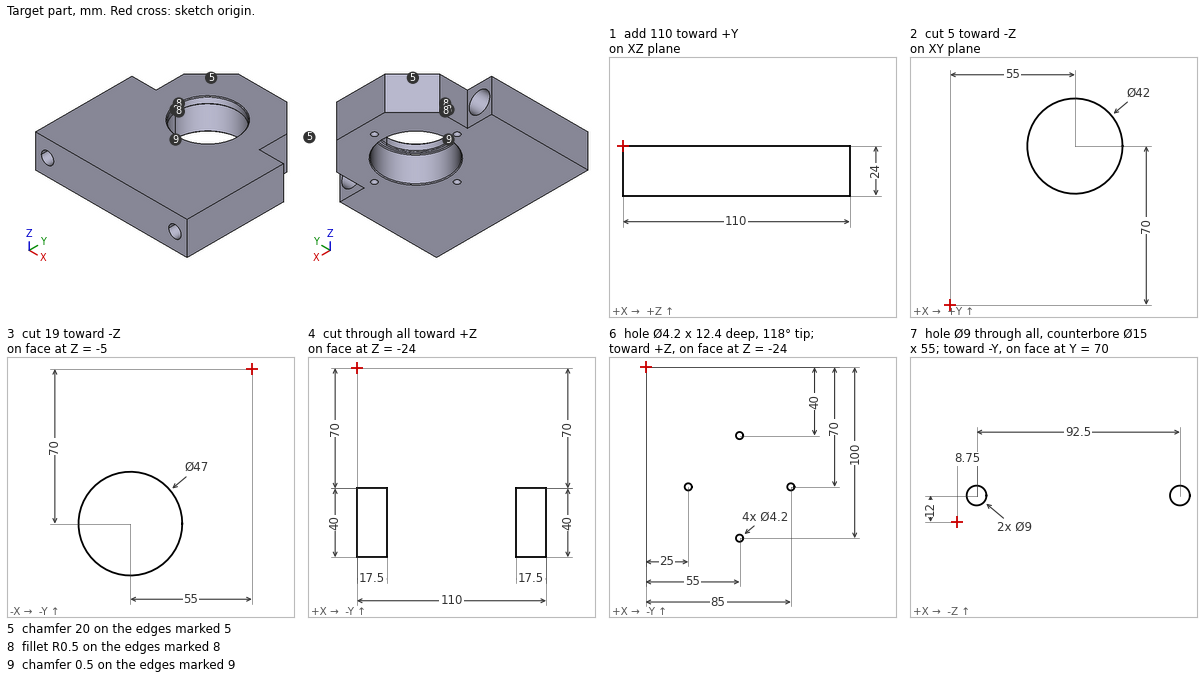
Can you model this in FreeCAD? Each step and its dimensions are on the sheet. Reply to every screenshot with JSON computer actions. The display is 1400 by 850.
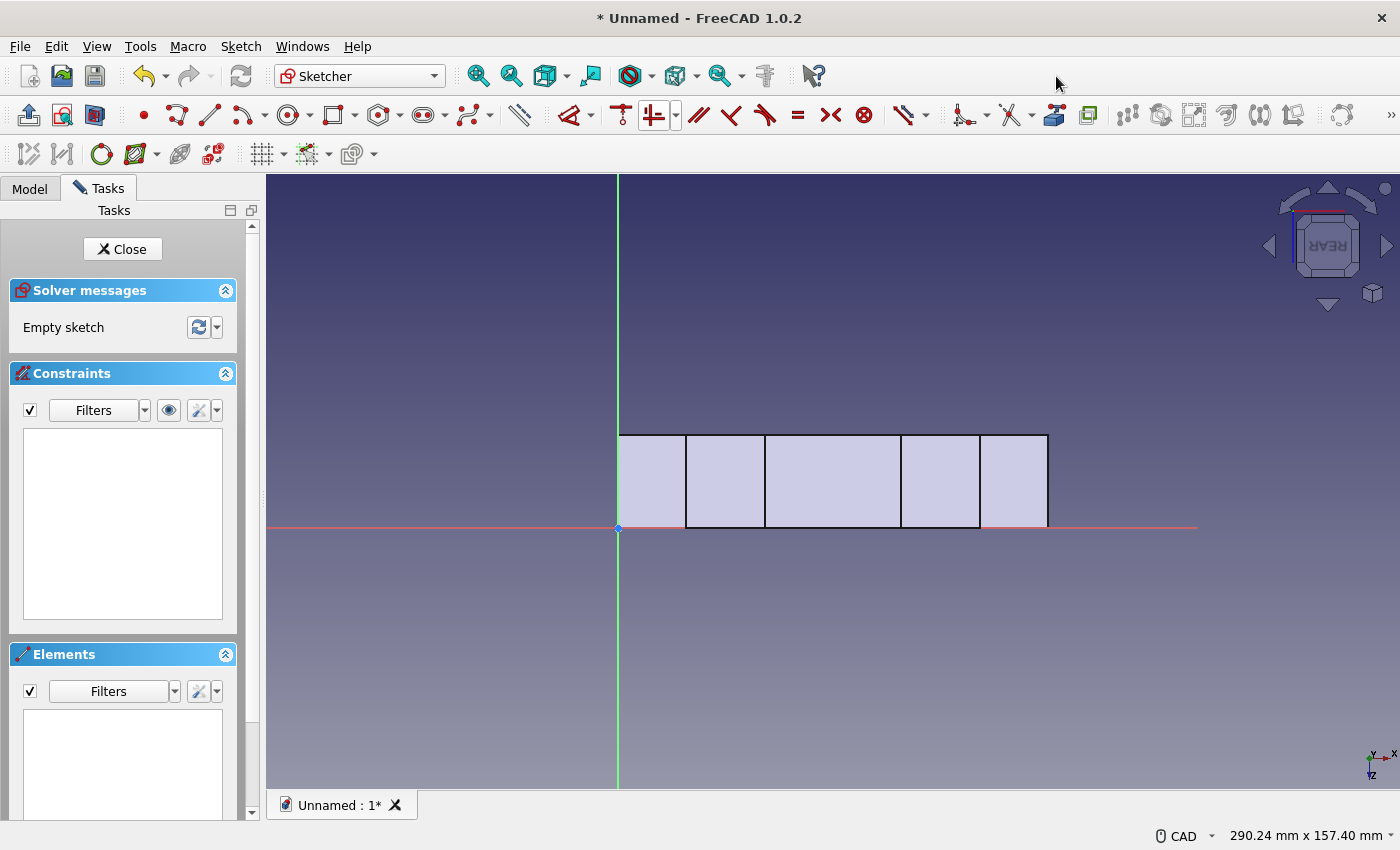
{"action": "scroll", "coordinate": [947, 526], "scroll_direction": "up", "scroll_amount": 2}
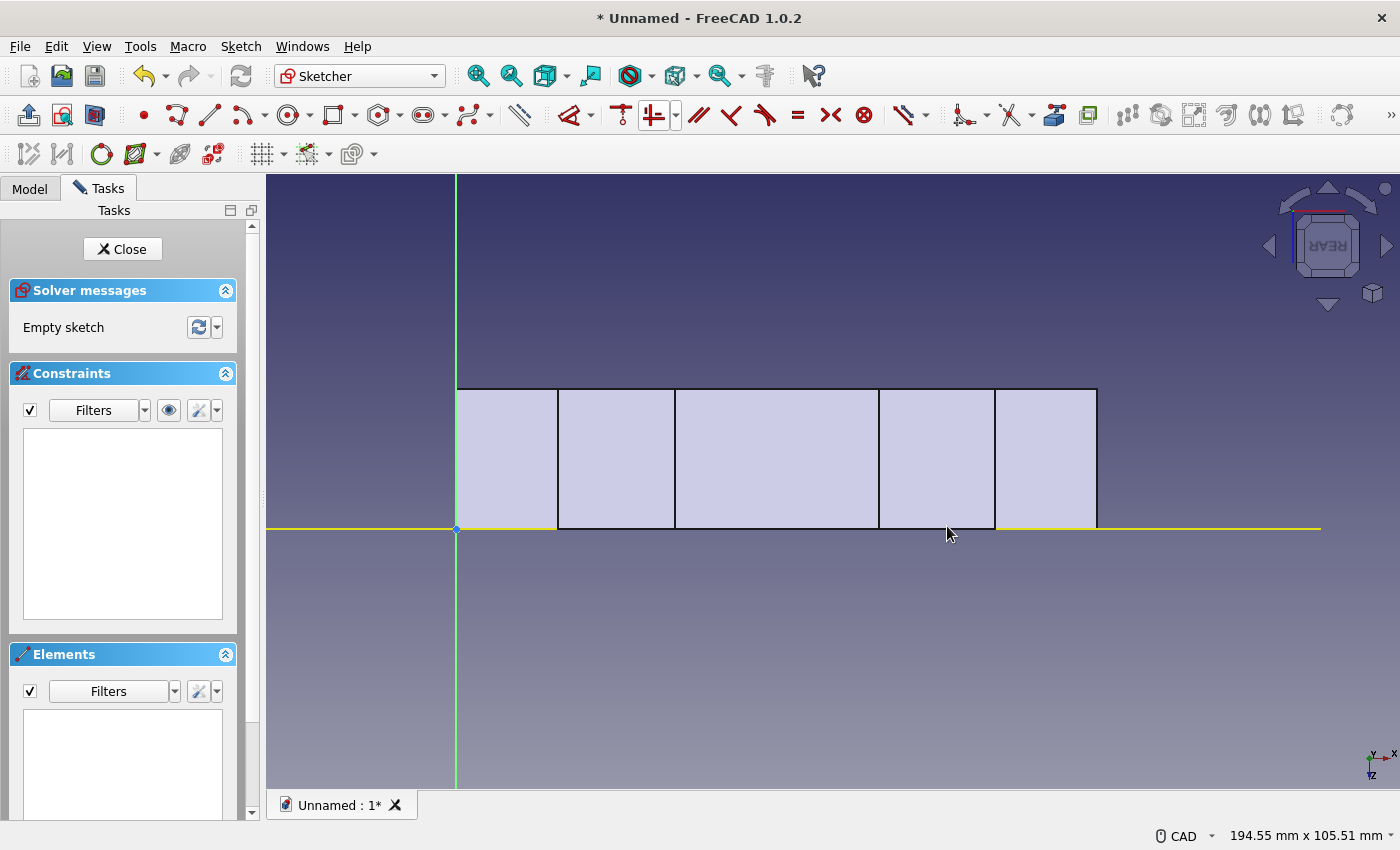
{"action": "left_click", "coordinate": [288, 116]}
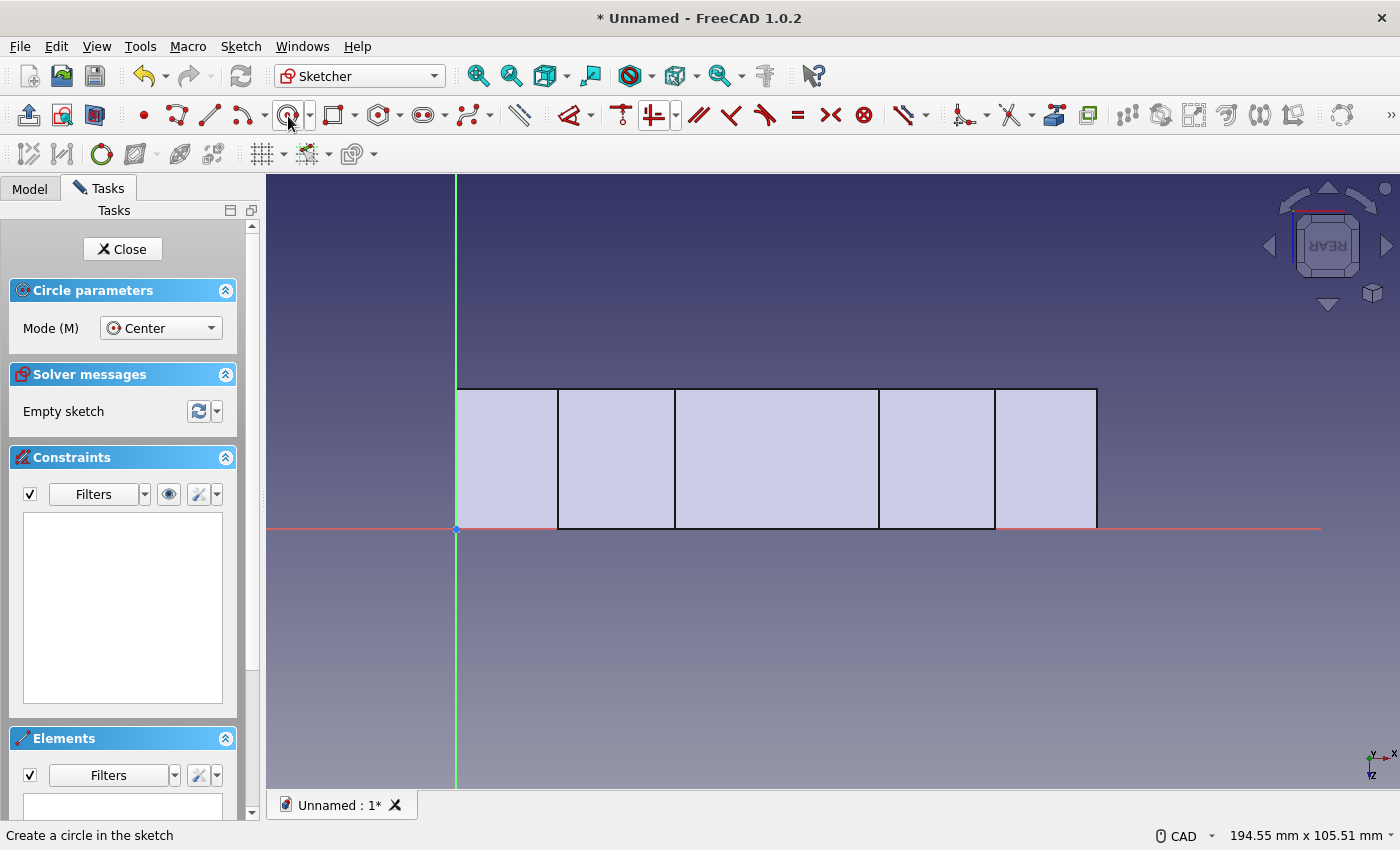
{"action": "left_click", "coordinate": [507, 459]}
{"action": "mouse_move", "coordinate": [526, 441]}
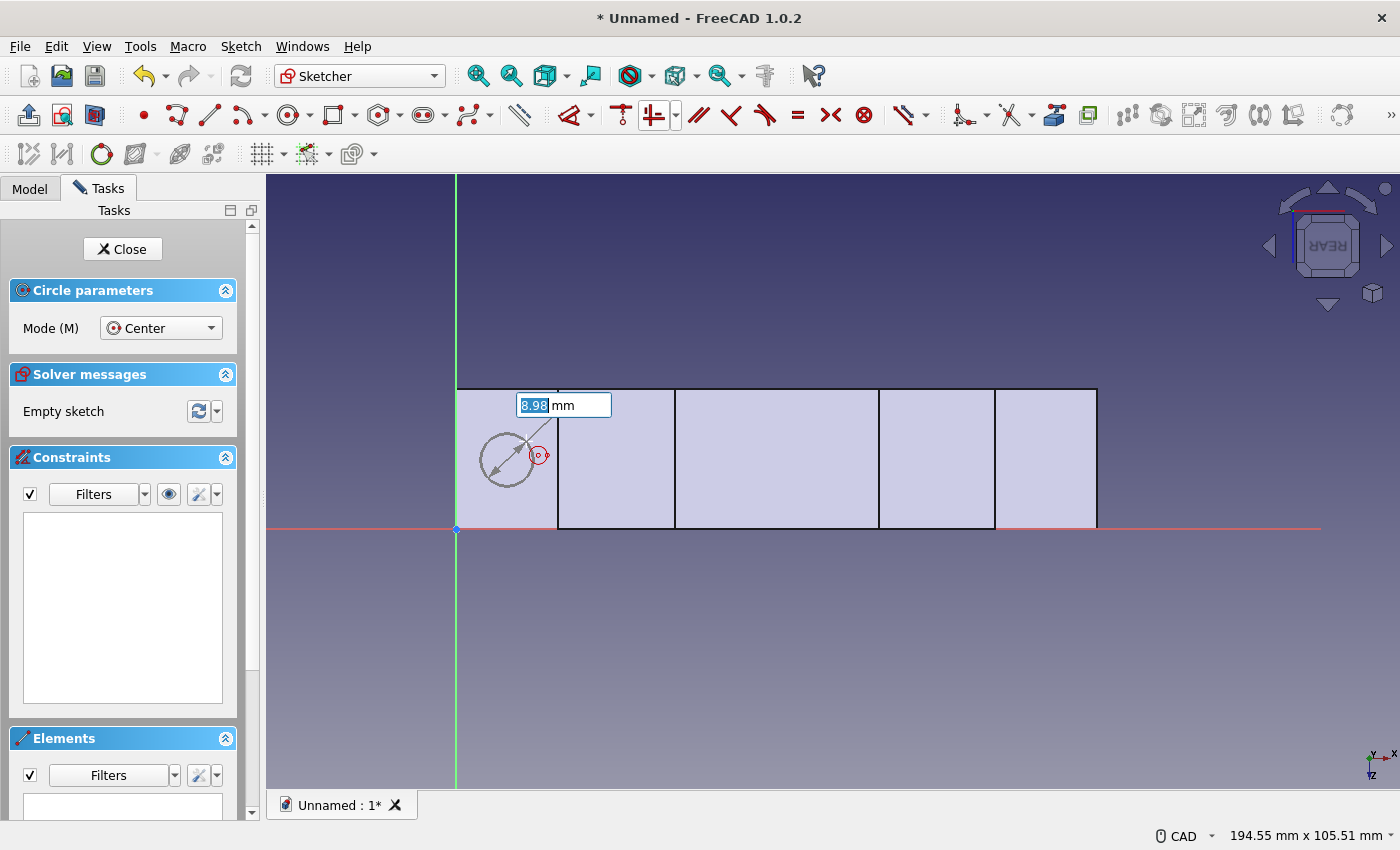
{"action": "type", "text": "9"}
{"action": "key", "text": "Return"}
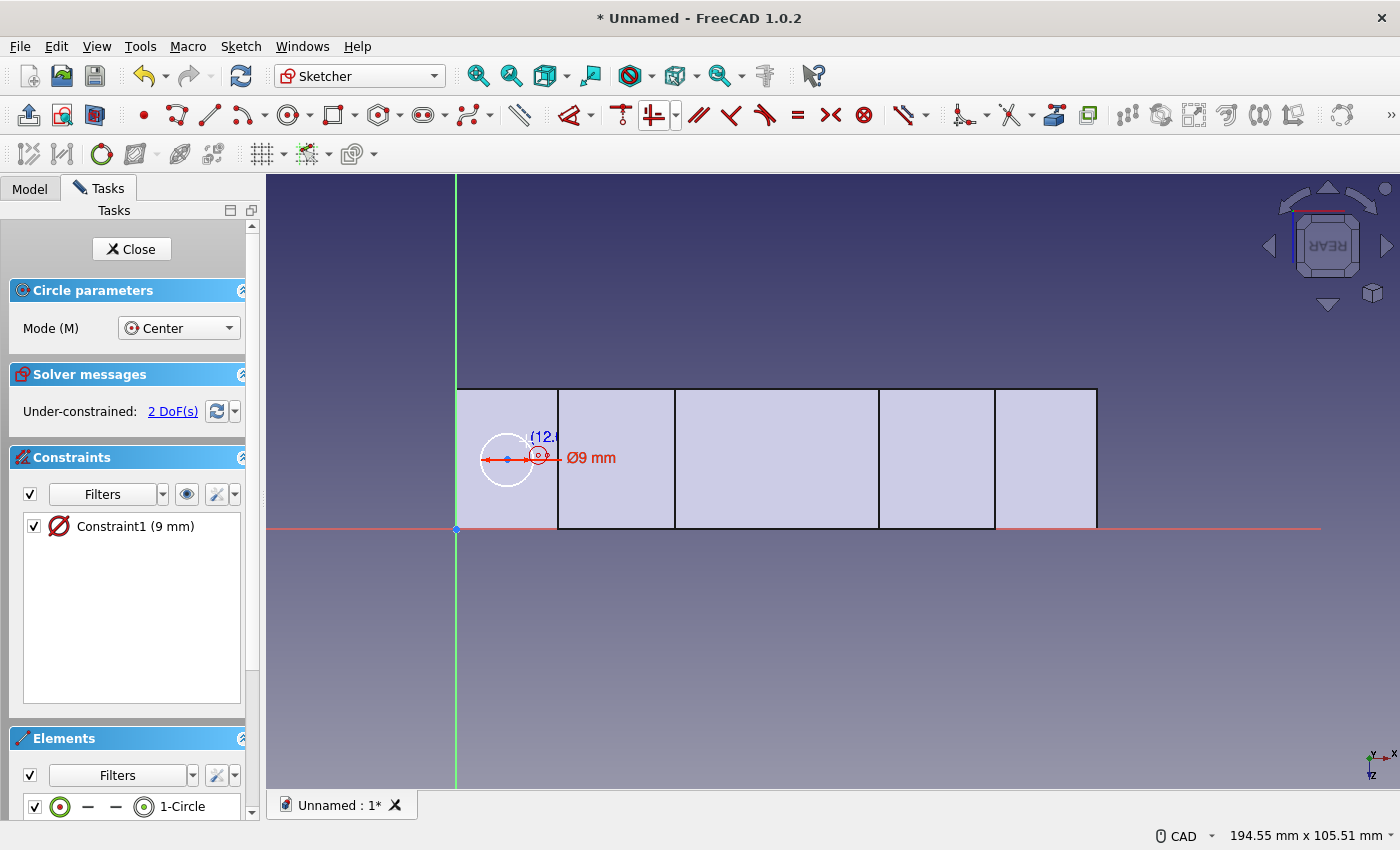
{"action": "left_click", "coordinate": [1046, 459]}
{"action": "mouse_move", "coordinate": [1065, 441]}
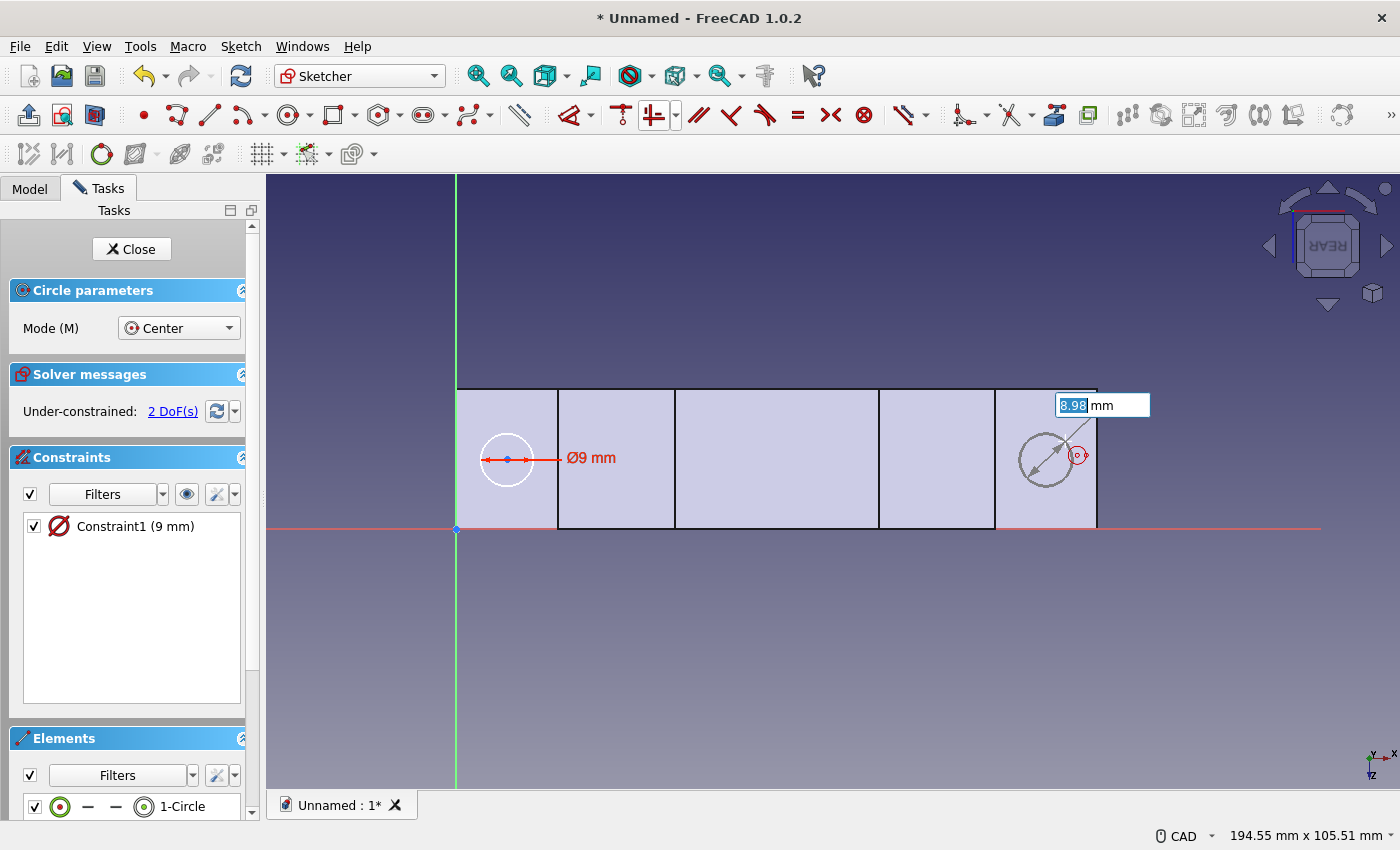
{"action": "type", "text": "9"}
{"action": "key", "text": "Return"}
{"action": "key", "text": "Escape"}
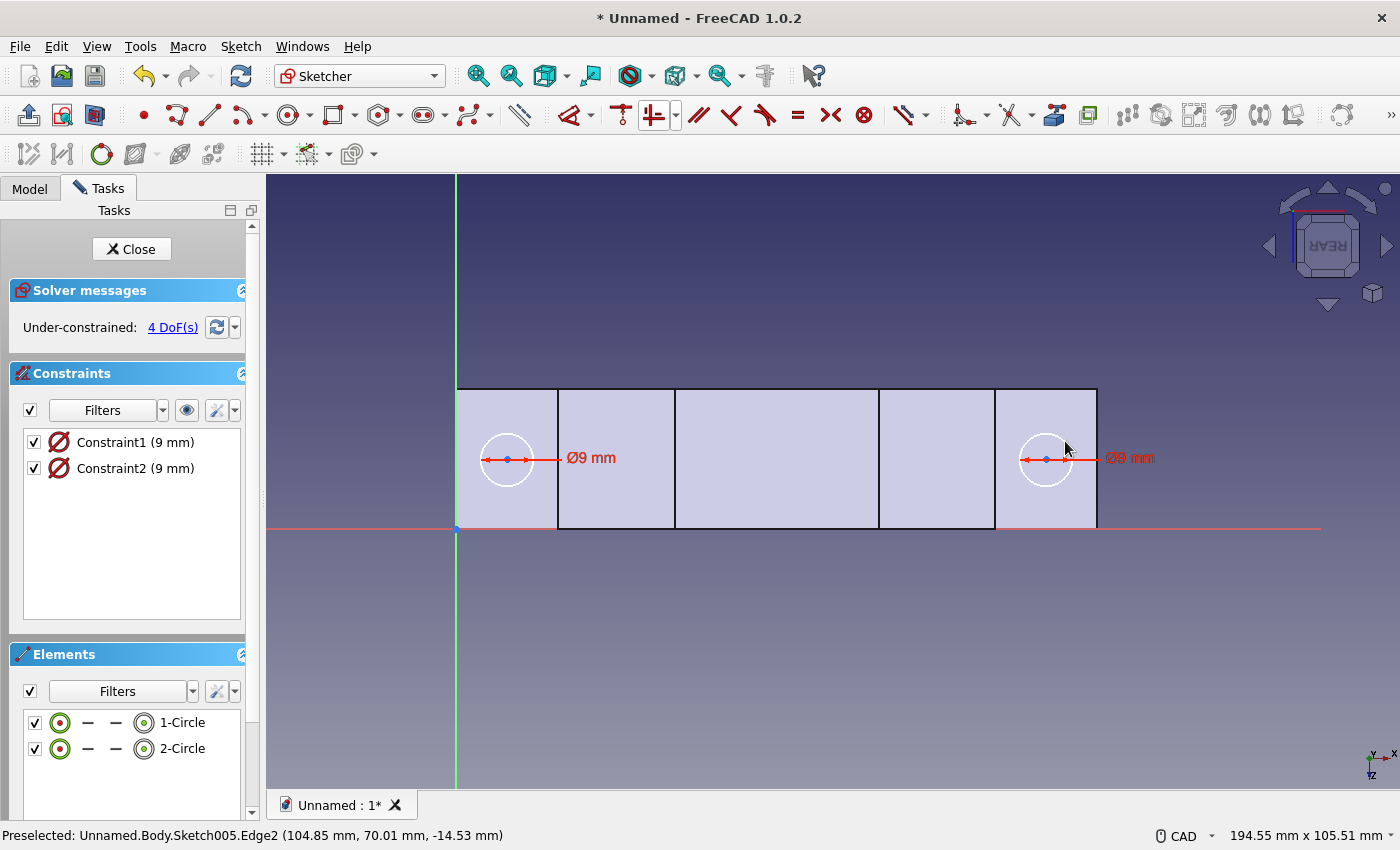
{"action": "left_click", "coordinate": [507, 460]}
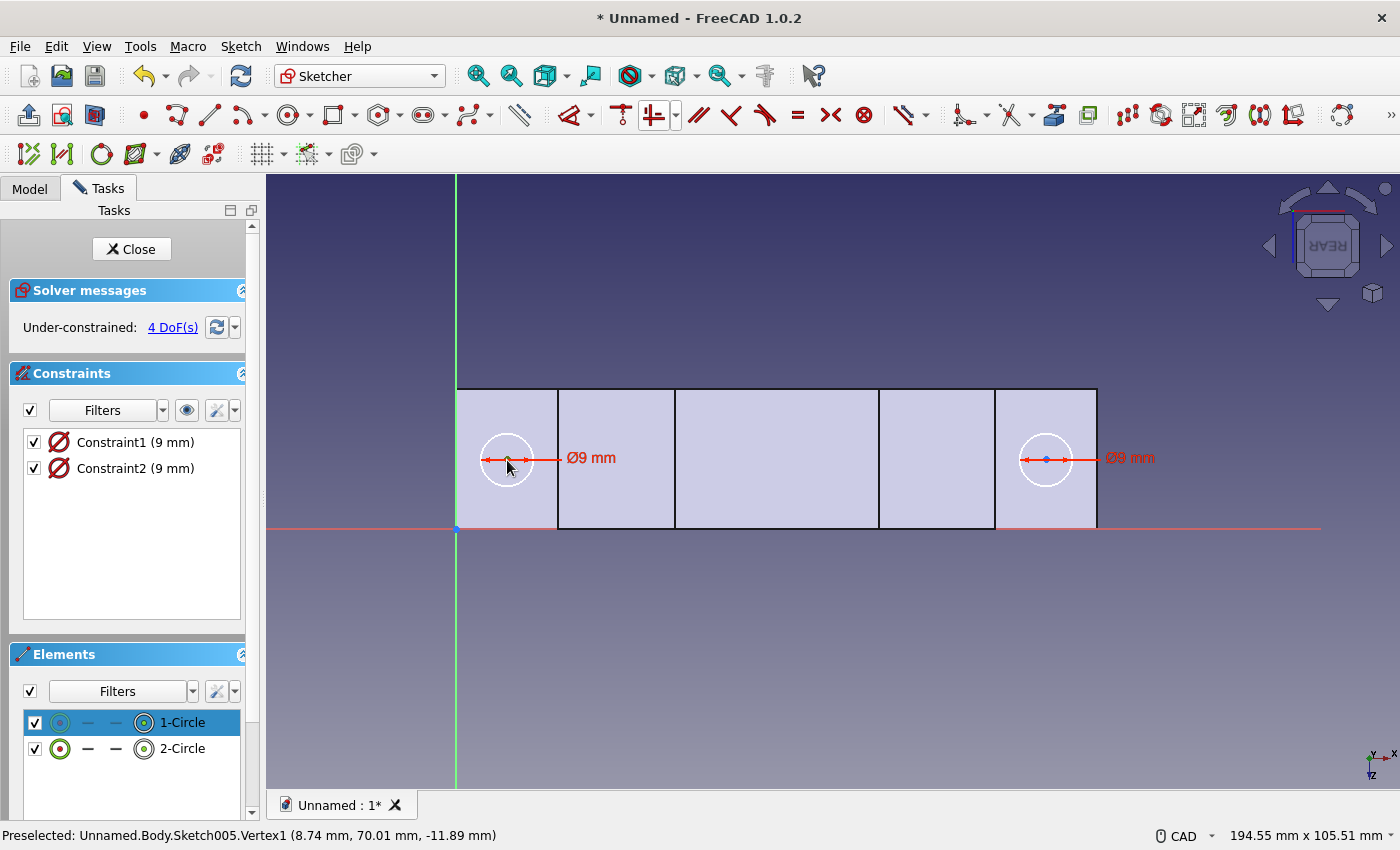
{"action": "left_click", "coordinate": [1046, 460]}